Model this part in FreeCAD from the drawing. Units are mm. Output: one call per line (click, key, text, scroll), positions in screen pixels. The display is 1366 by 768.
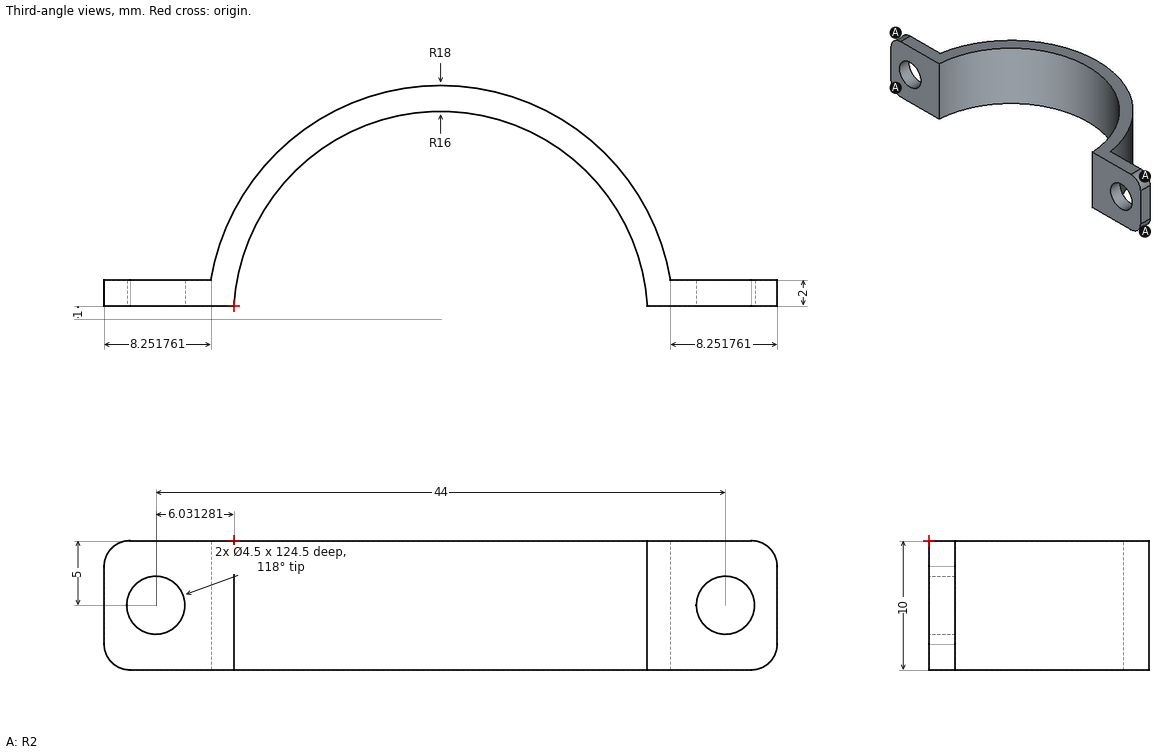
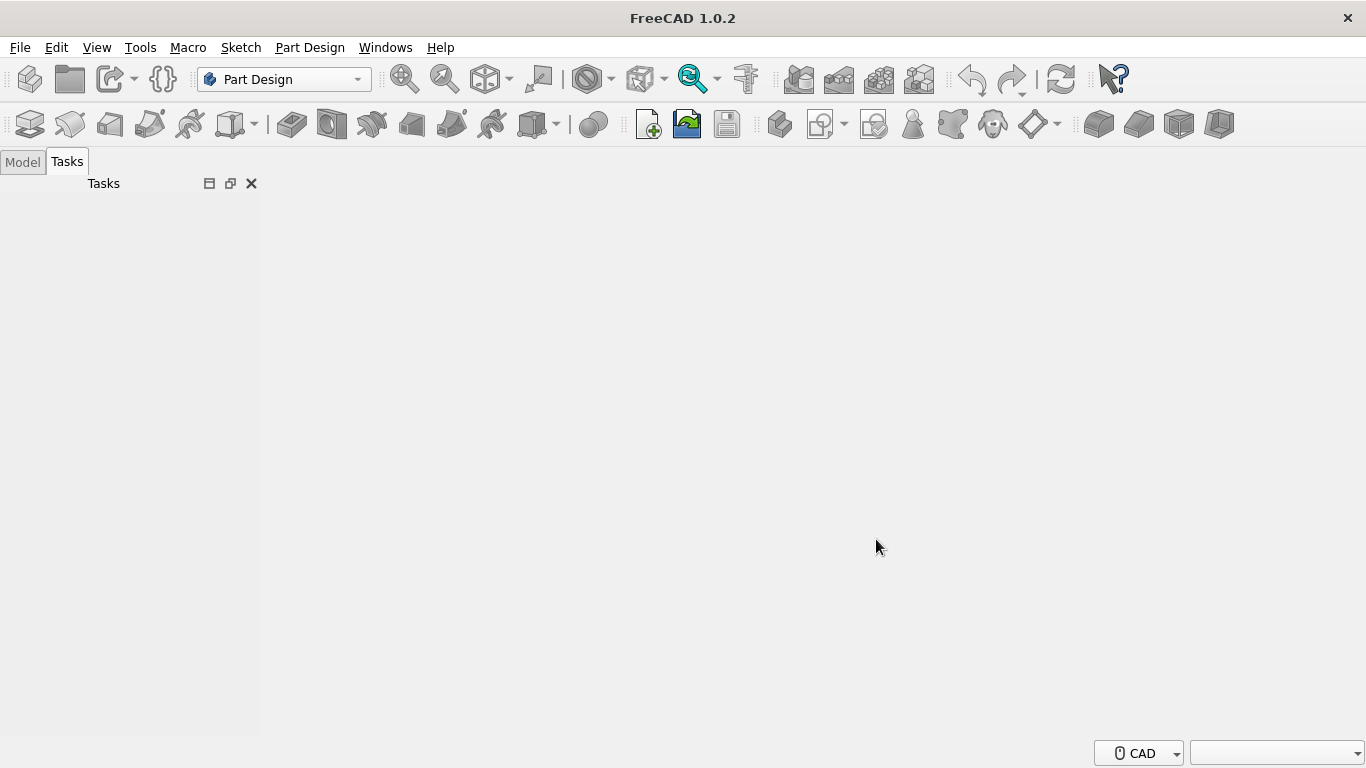
click(648, 124)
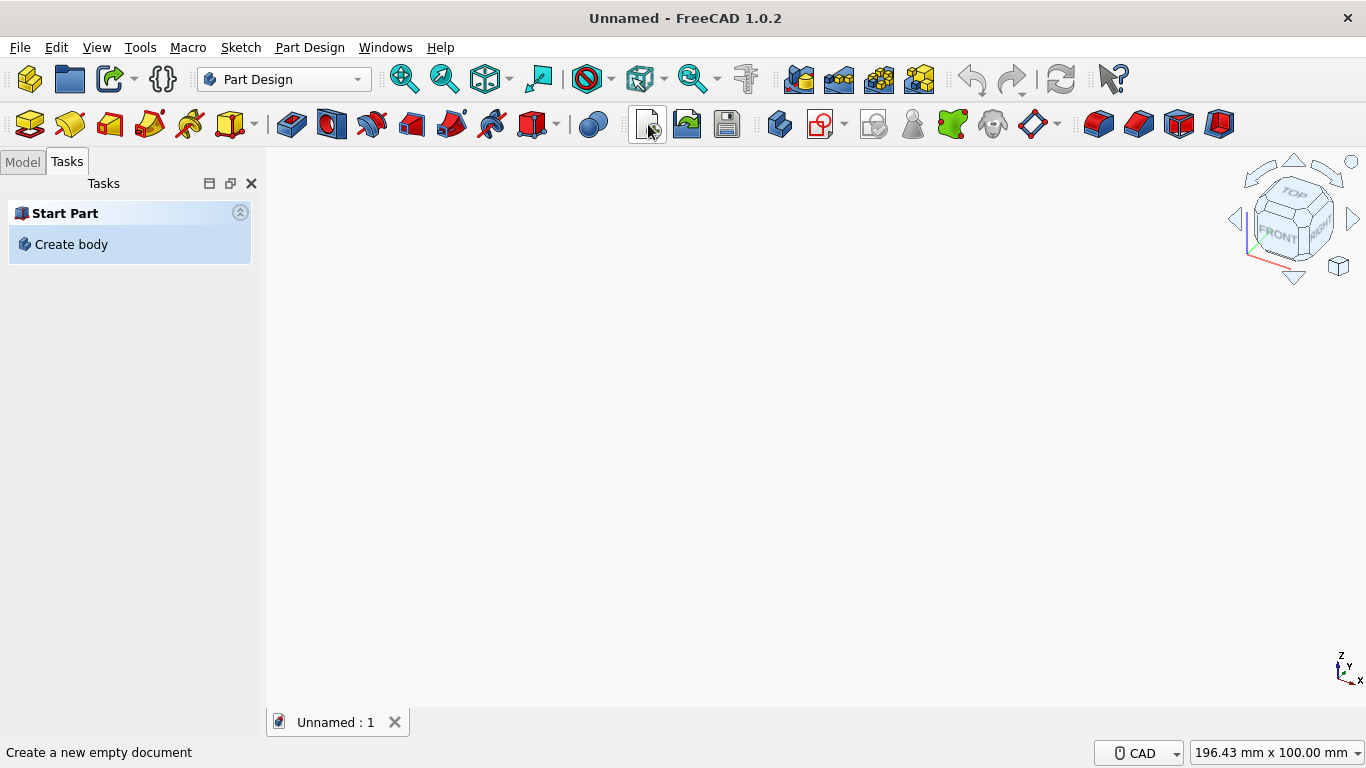
click(820, 124)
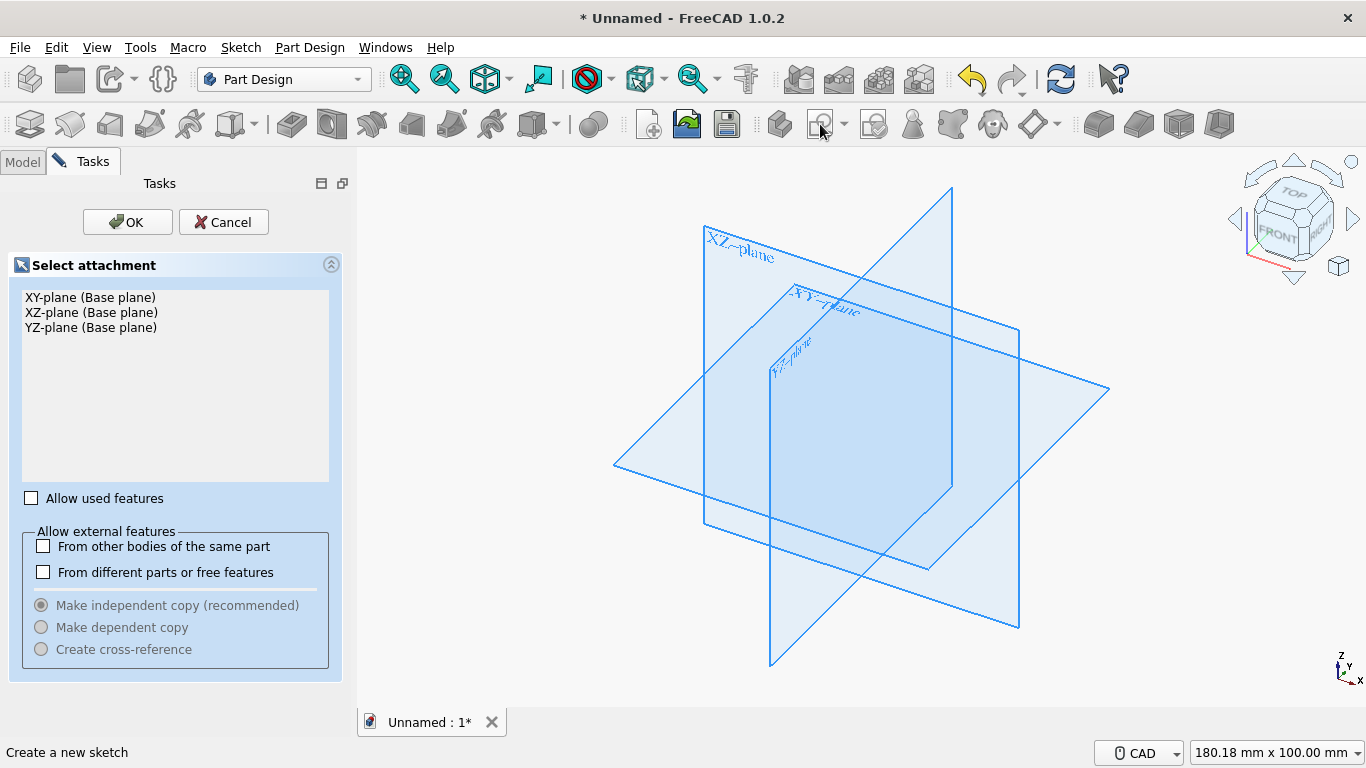
click(82, 298)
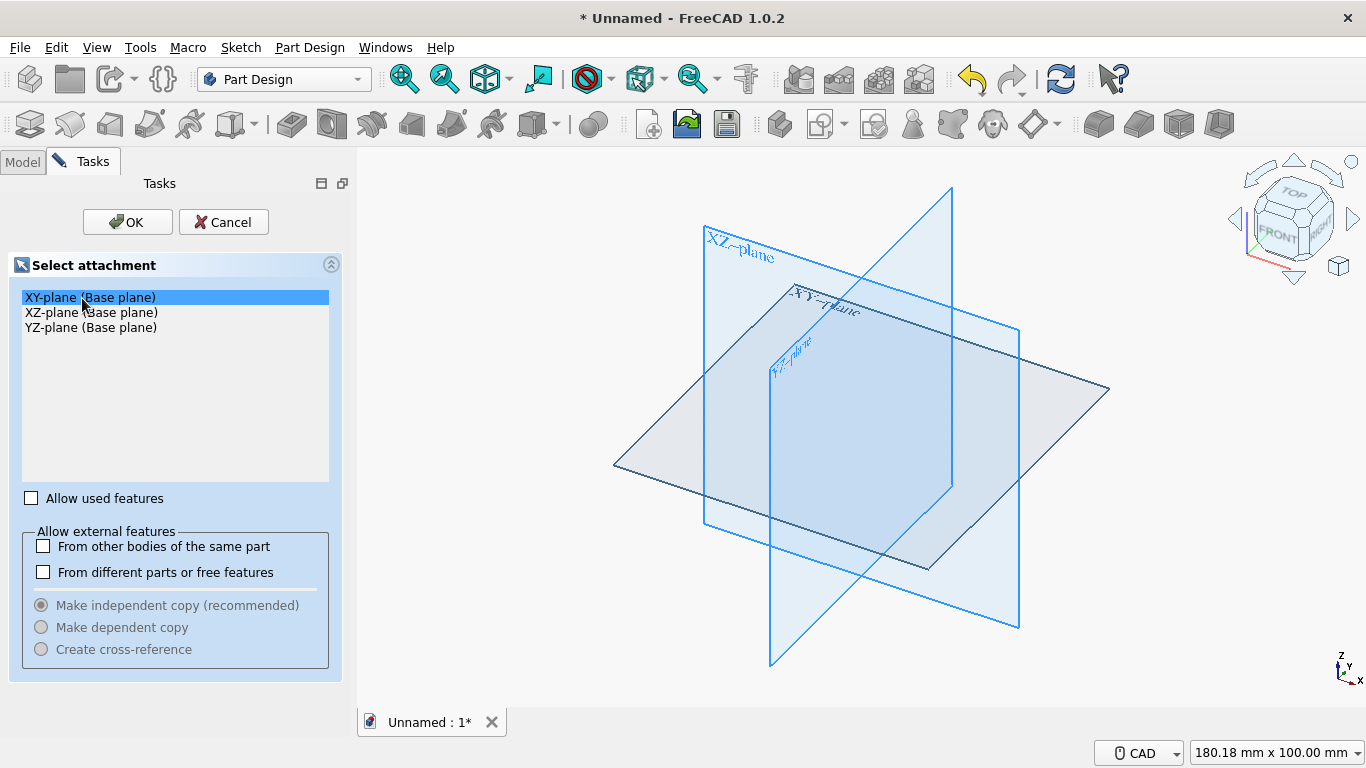
click(128, 222)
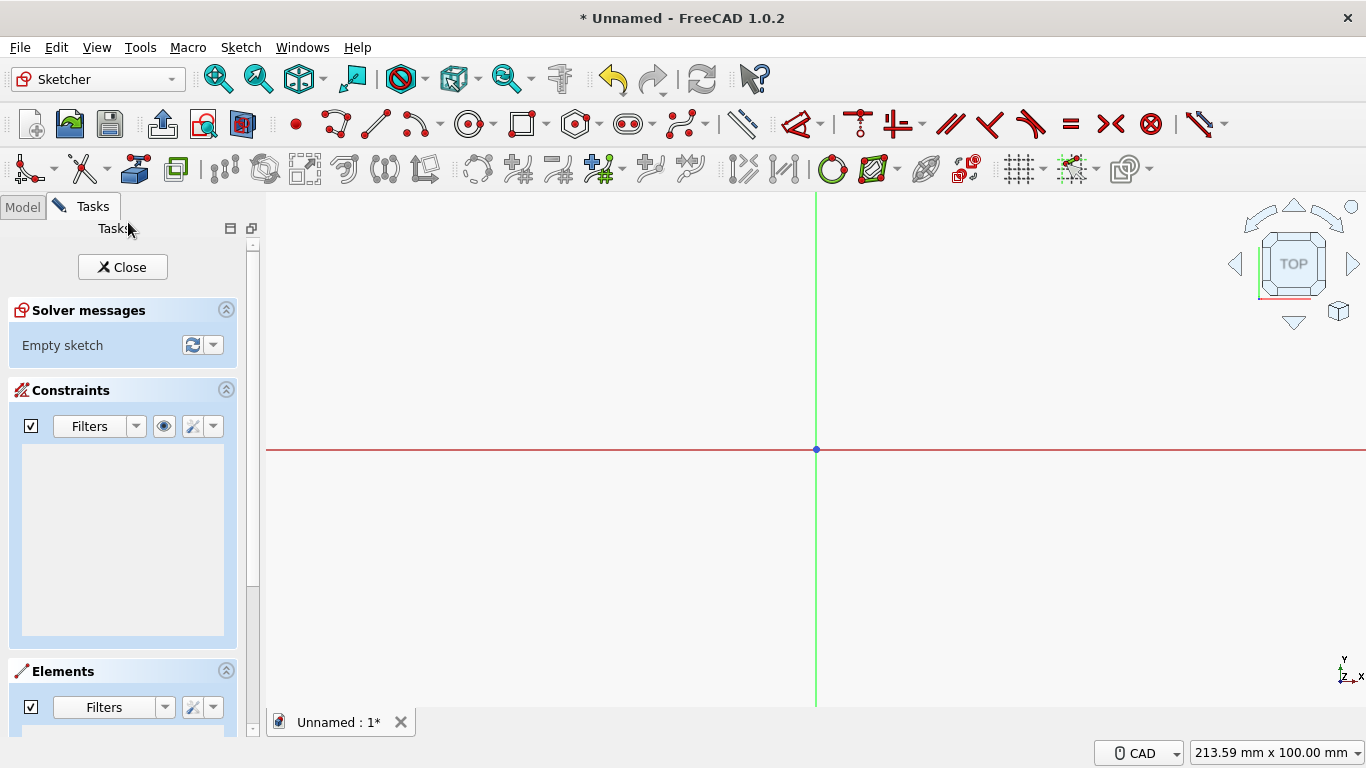
scroll(1021, 370, up, 4)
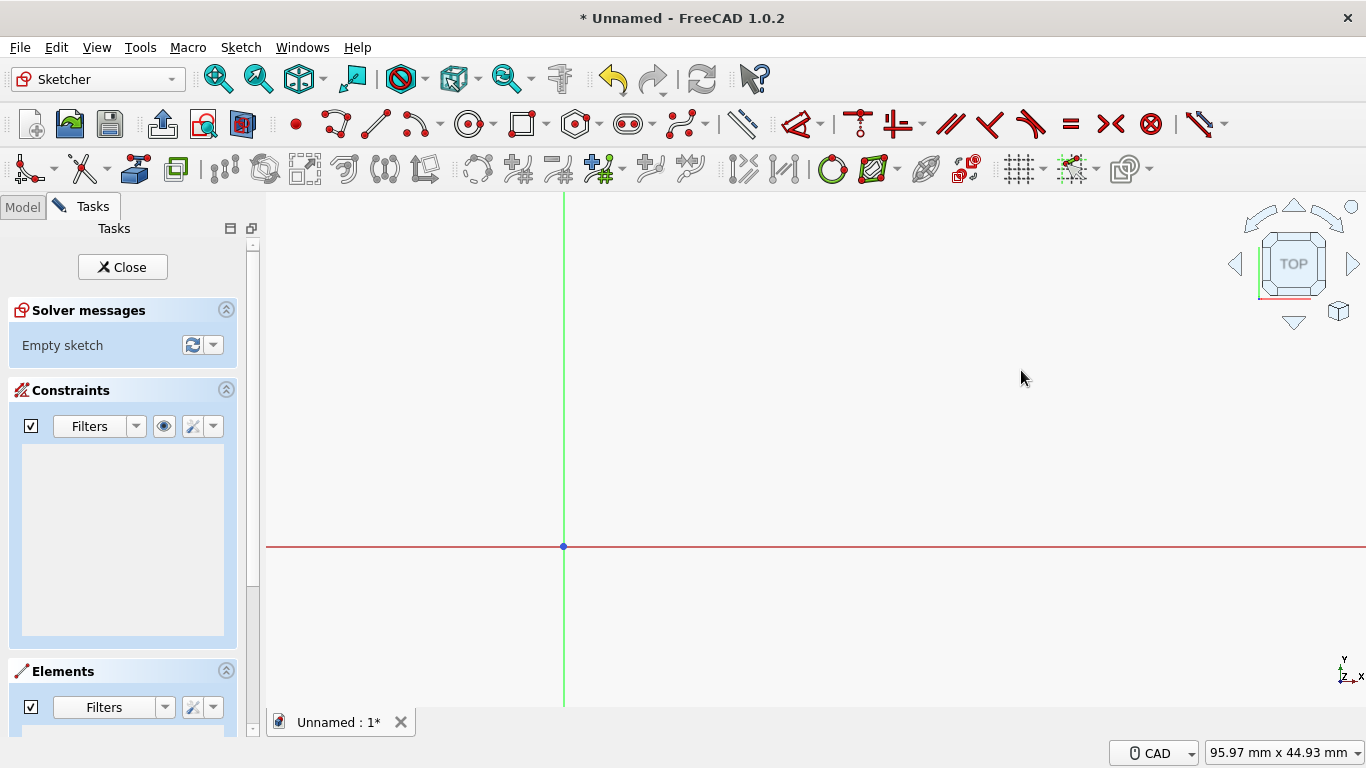
click(336, 124)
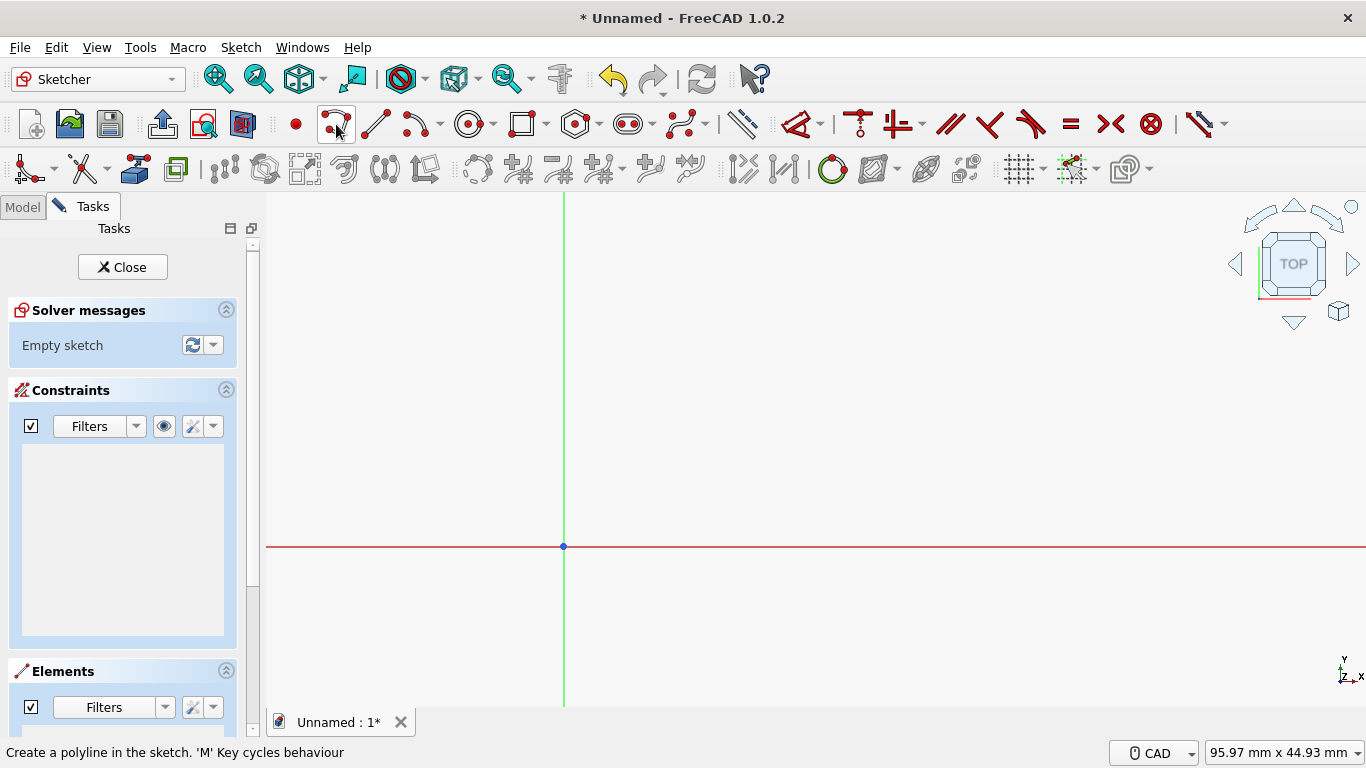
click(930, 547)
click(1045, 538)
click(1045, 524)
click(950, 524)
right_click(950, 524)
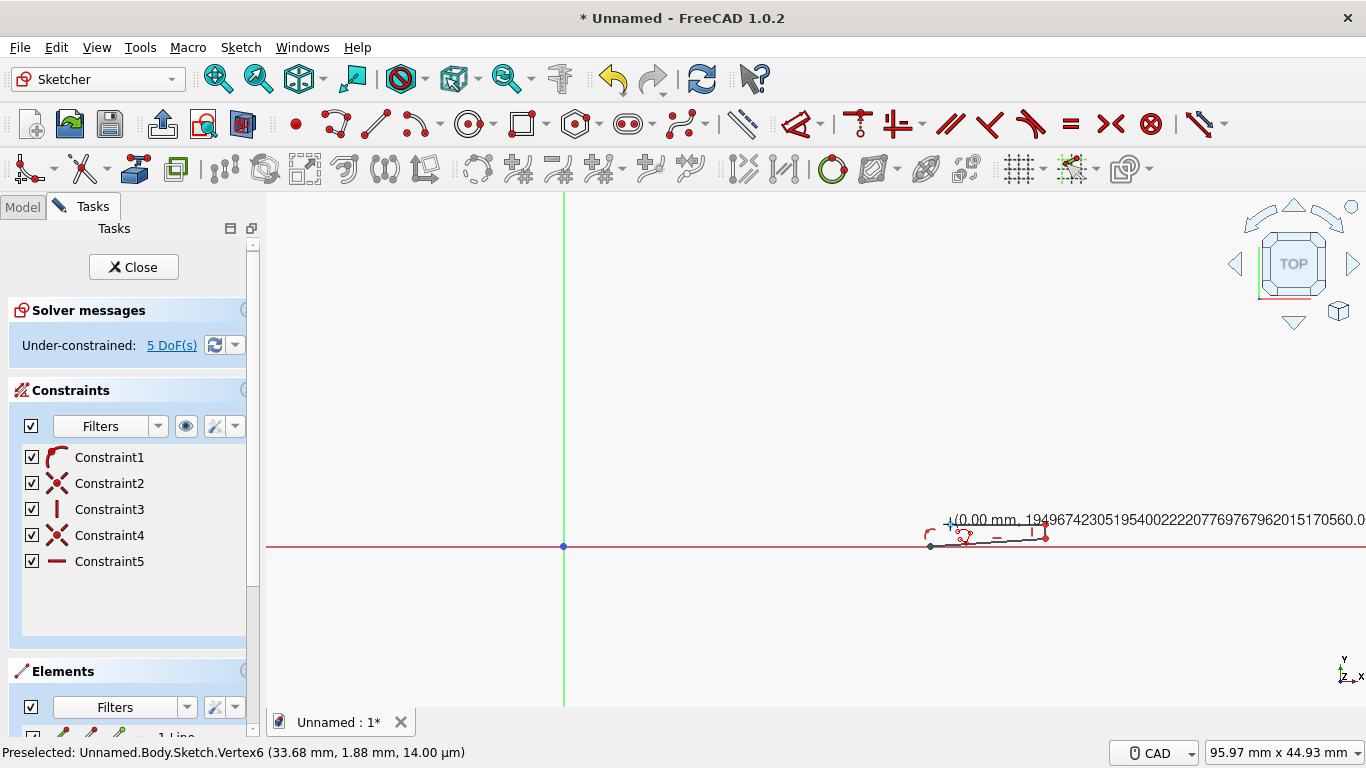
click(544, 524)
click(449, 524)
click(449, 547)
click(564, 547)
right_click(564, 547)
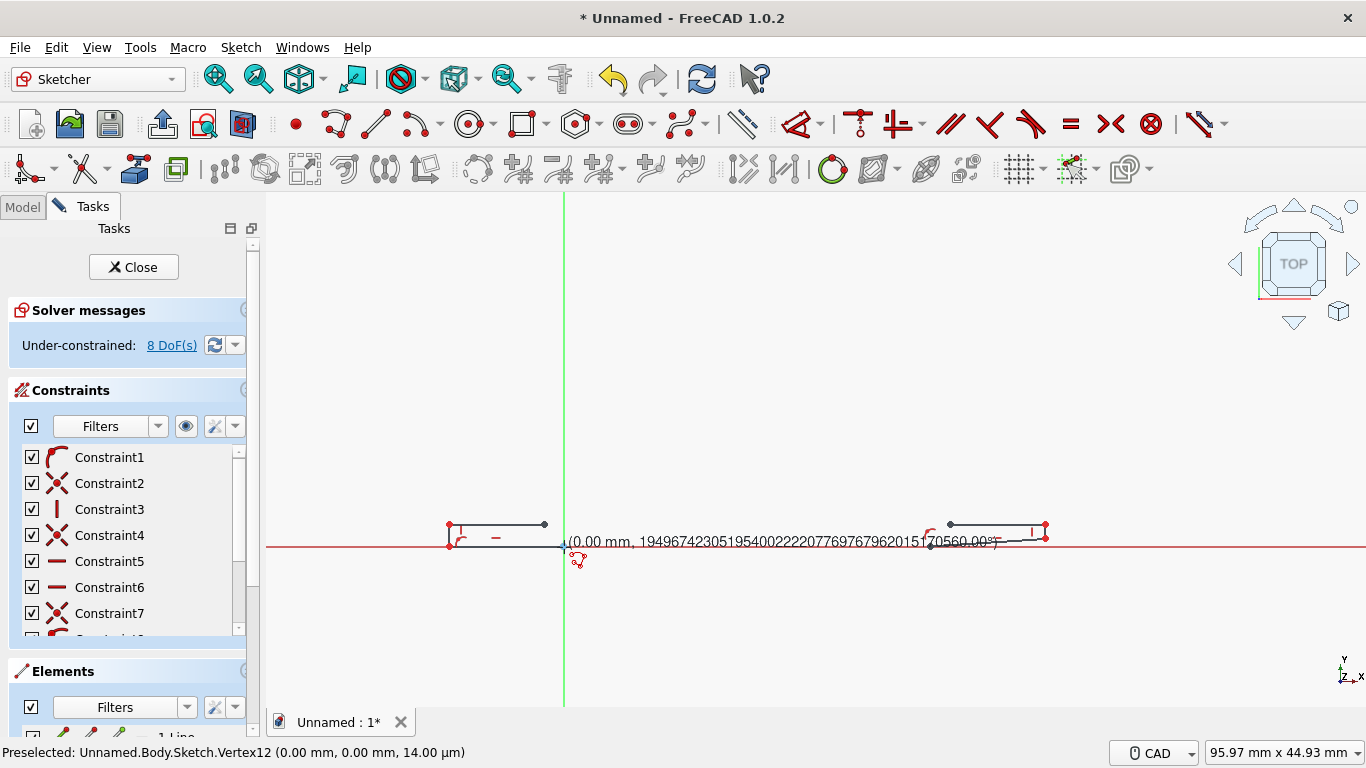
key(g)
key(3)
key(a)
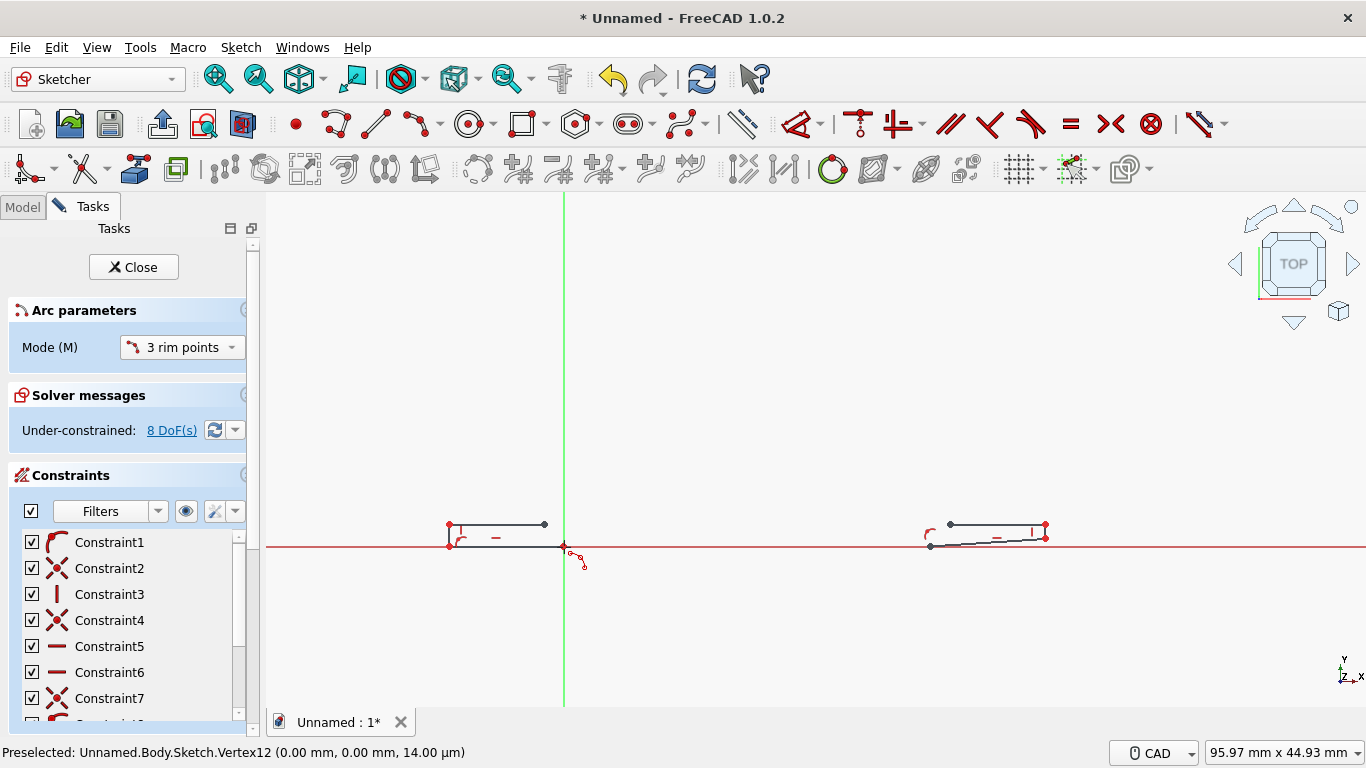
click(950, 525)
click(544, 525)
click(747, 352)